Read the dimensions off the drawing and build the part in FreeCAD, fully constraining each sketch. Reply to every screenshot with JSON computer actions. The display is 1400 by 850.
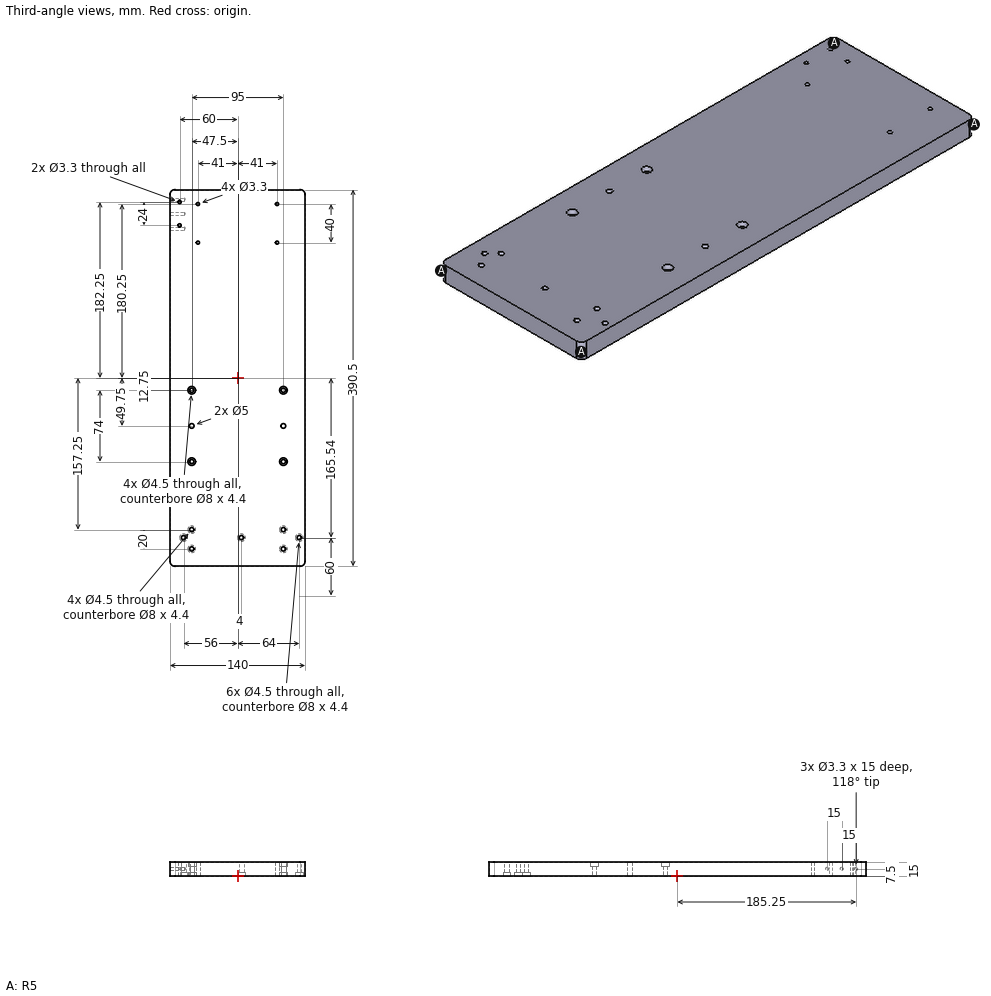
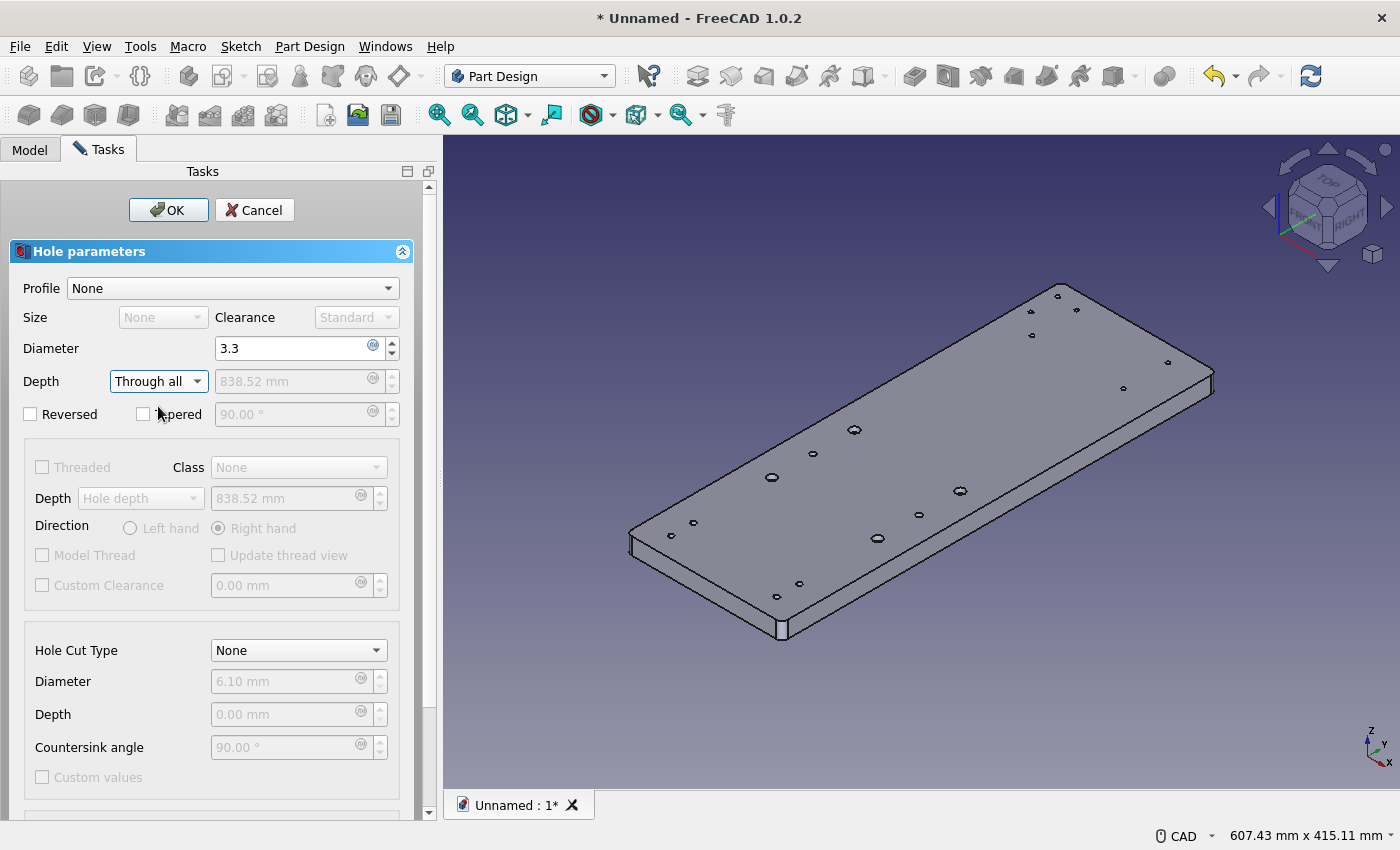
{"action": "left_click", "coordinate": [169, 210]}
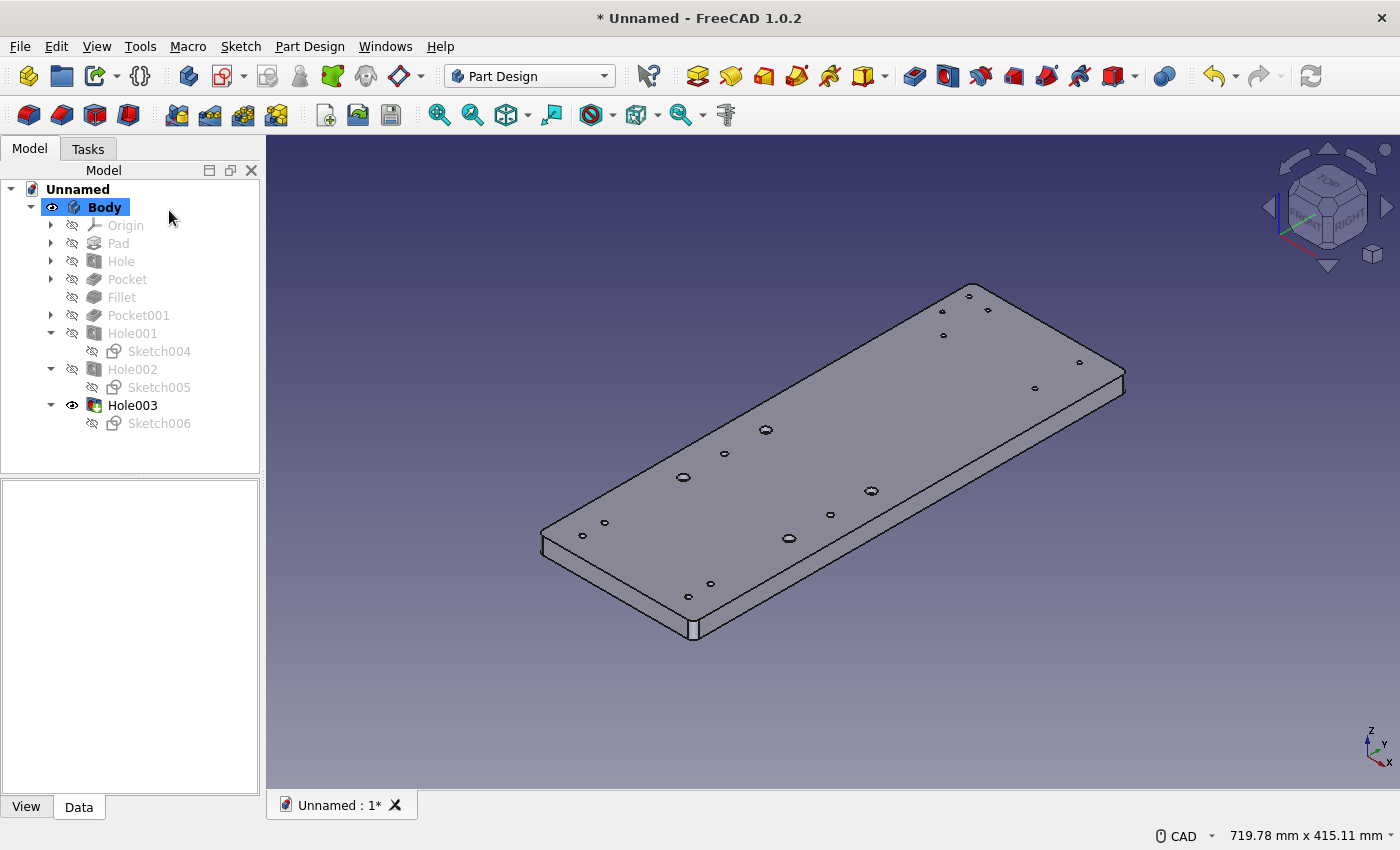
{"action": "key", "text": "5"}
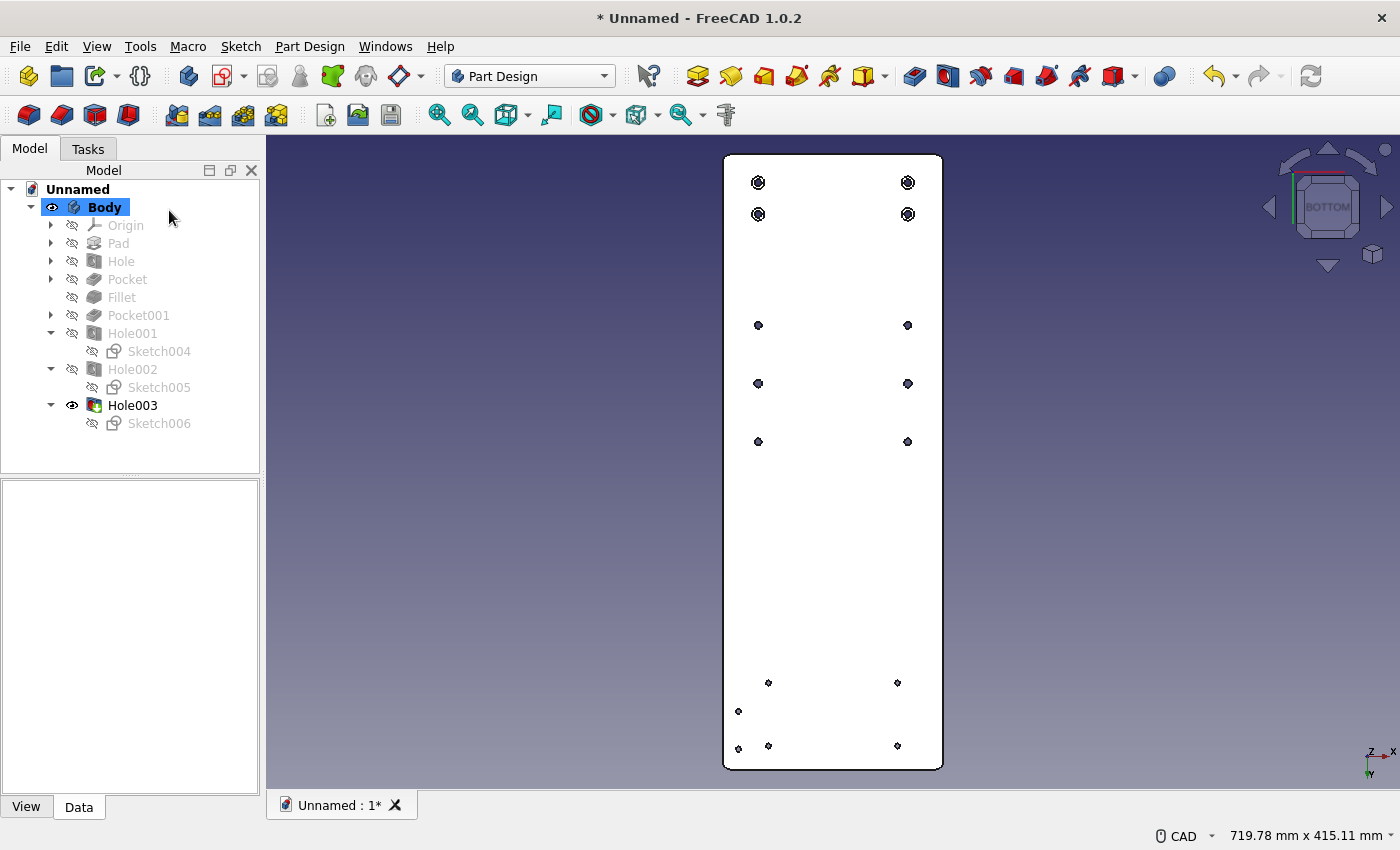
{"action": "left_click", "coordinate": [833, 549]}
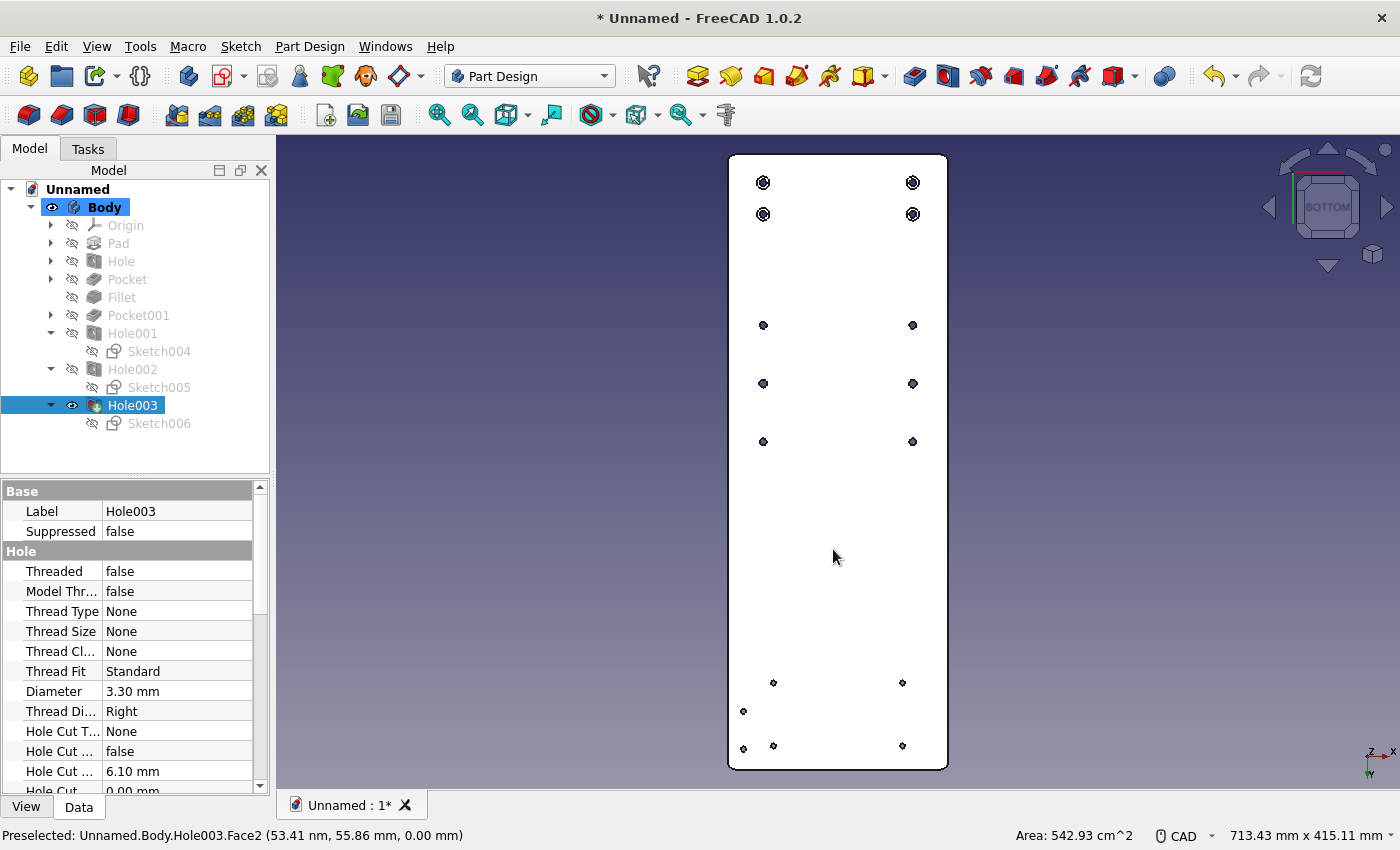
{"action": "left_click", "coordinate": [222, 76]}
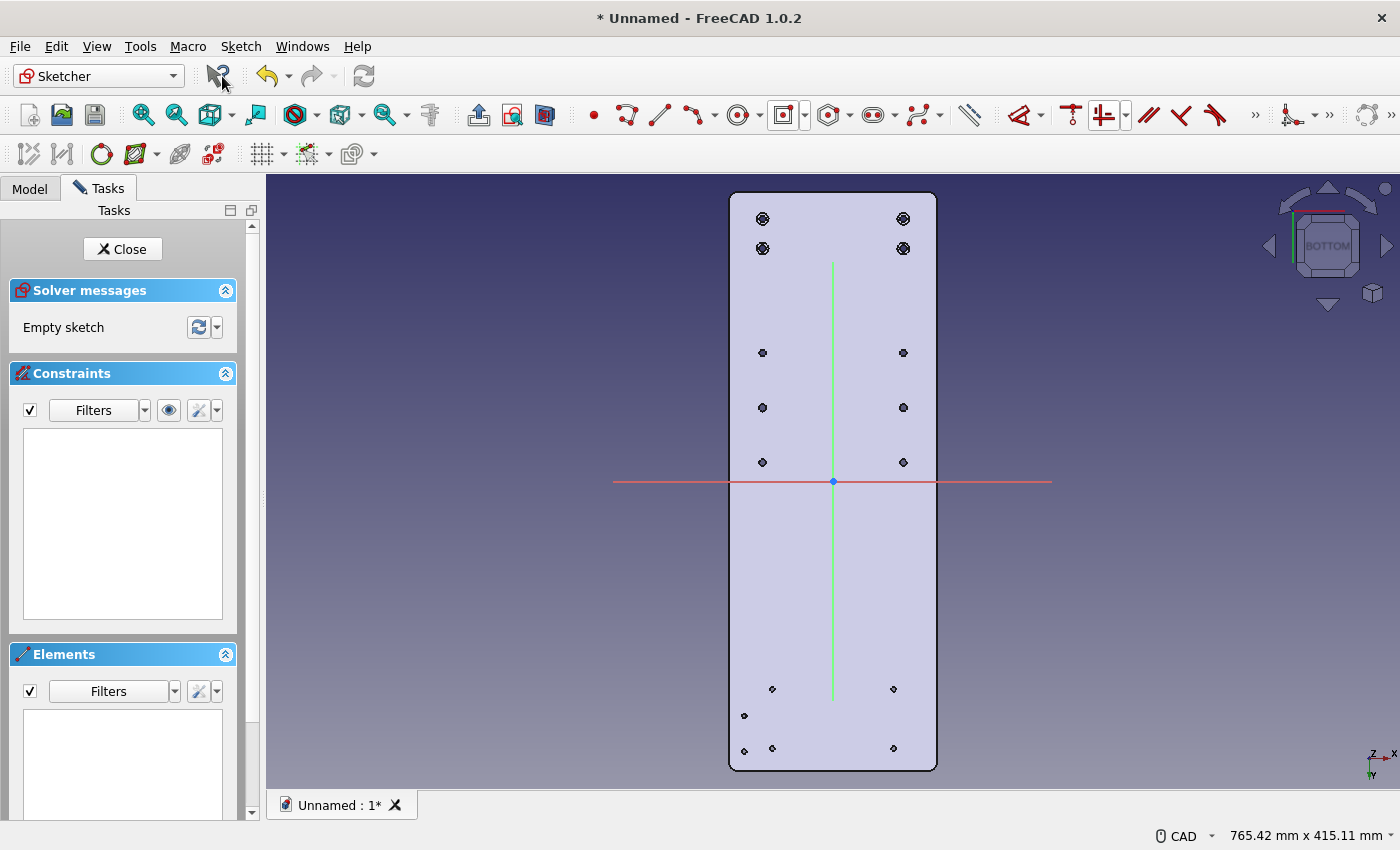
{"action": "scroll", "coordinate": [428, 761], "scroll_direction": "down", "scroll_amount": 1}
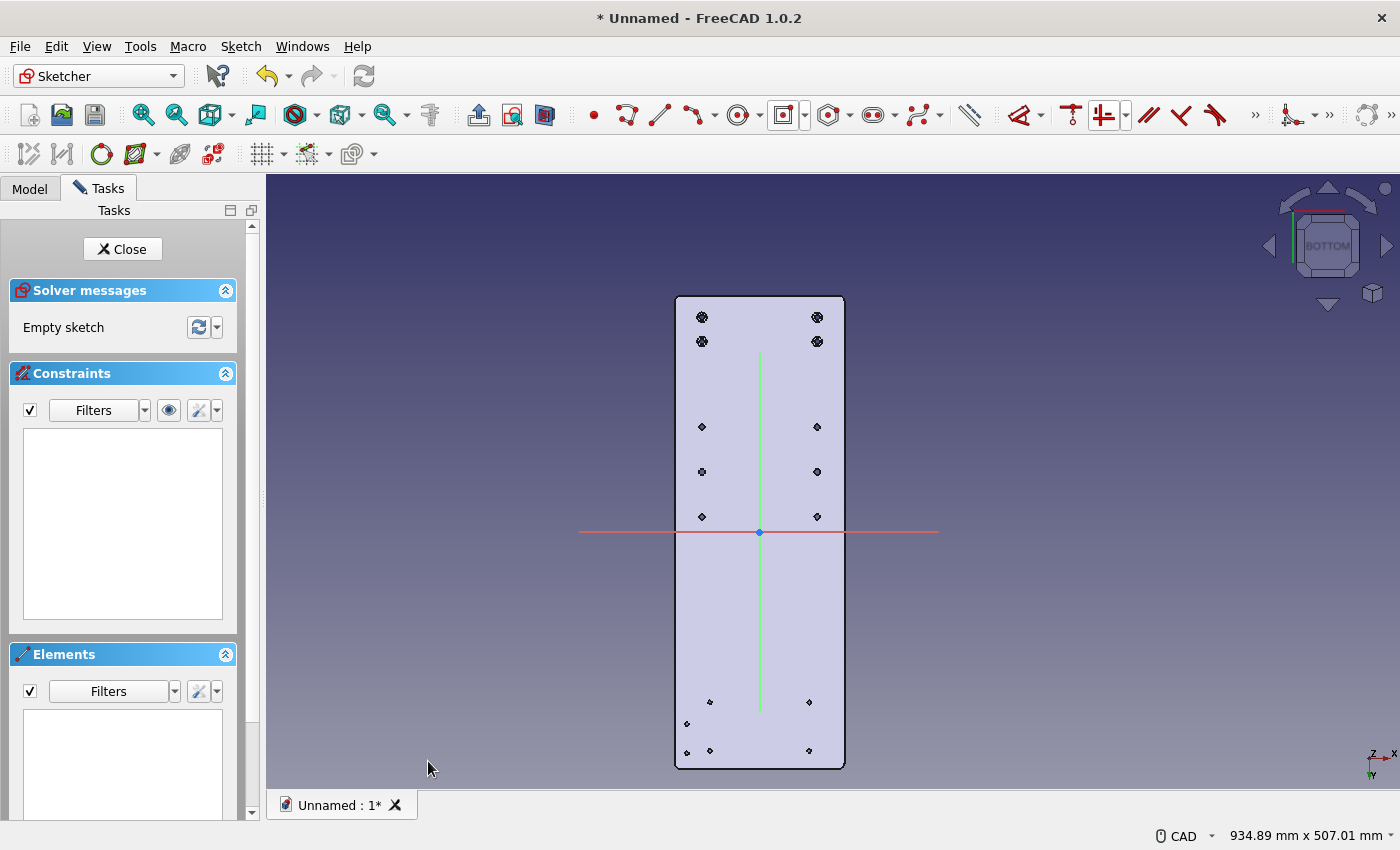
{"action": "scroll", "coordinate": [764, 217], "scroll_direction": "up", "scroll_amount": 2}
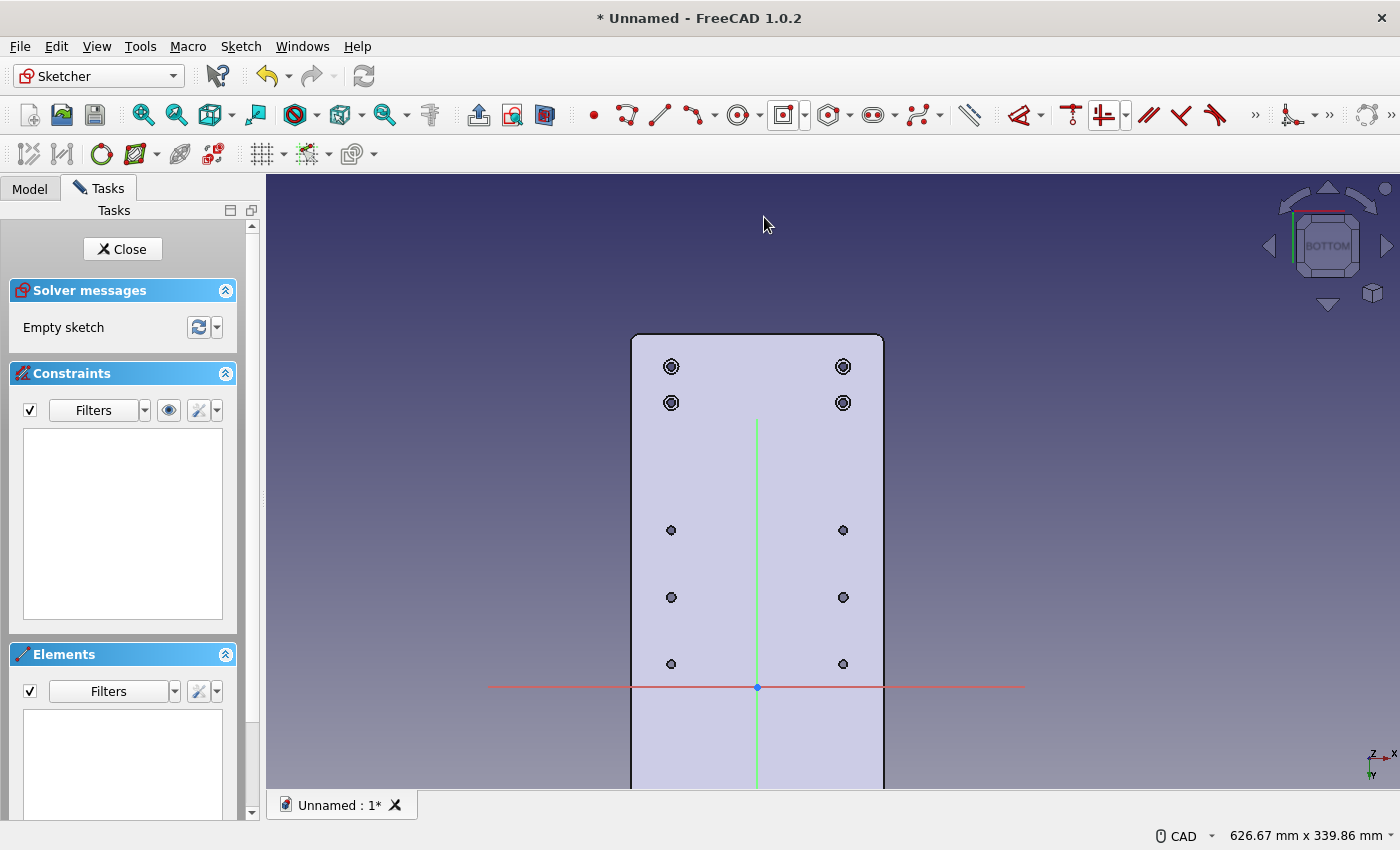
{"action": "left_click", "coordinate": [738, 116]}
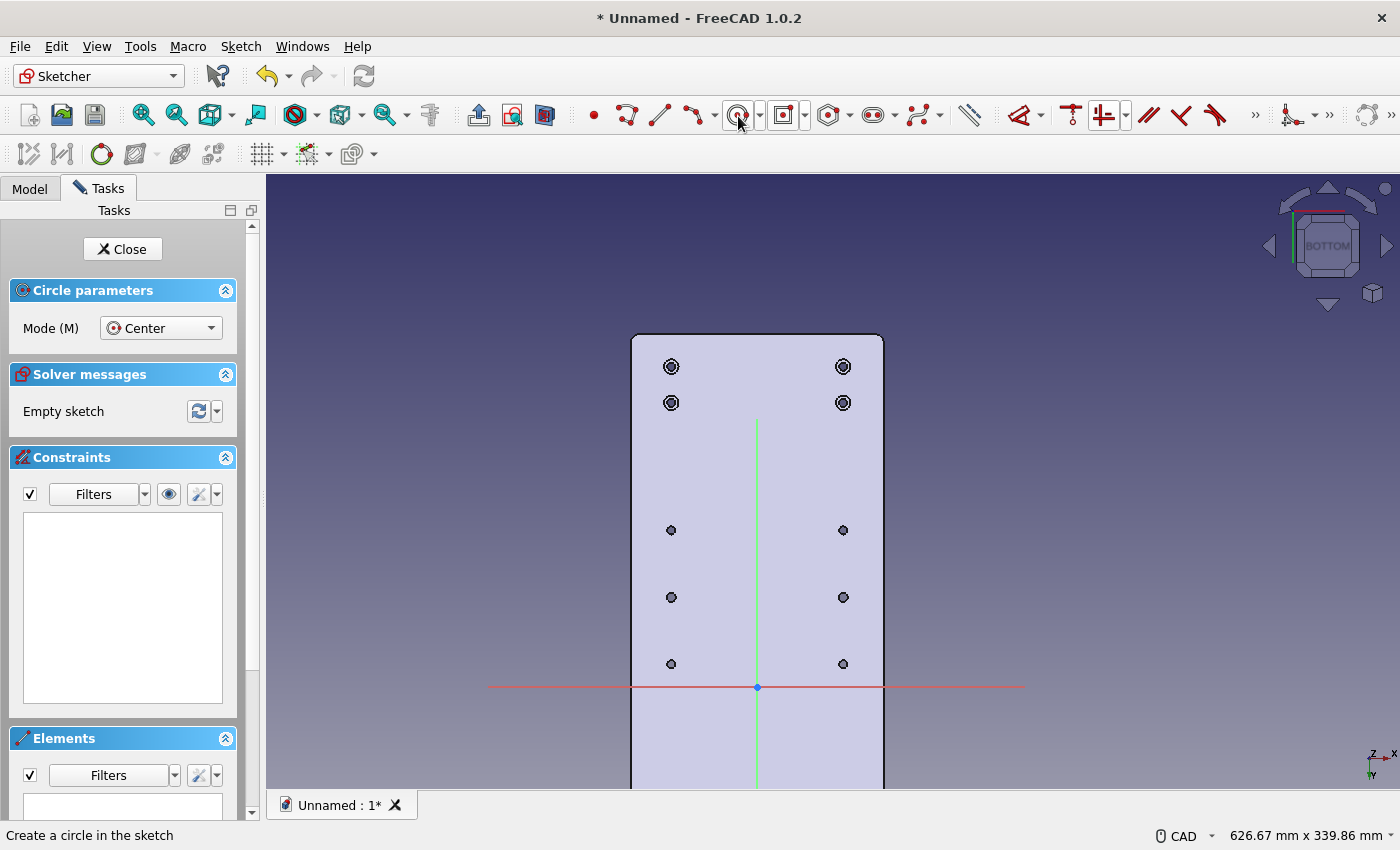
{"action": "scroll", "coordinate": [873, 388], "scroll_direction": "up", "scroll_amount": 9}